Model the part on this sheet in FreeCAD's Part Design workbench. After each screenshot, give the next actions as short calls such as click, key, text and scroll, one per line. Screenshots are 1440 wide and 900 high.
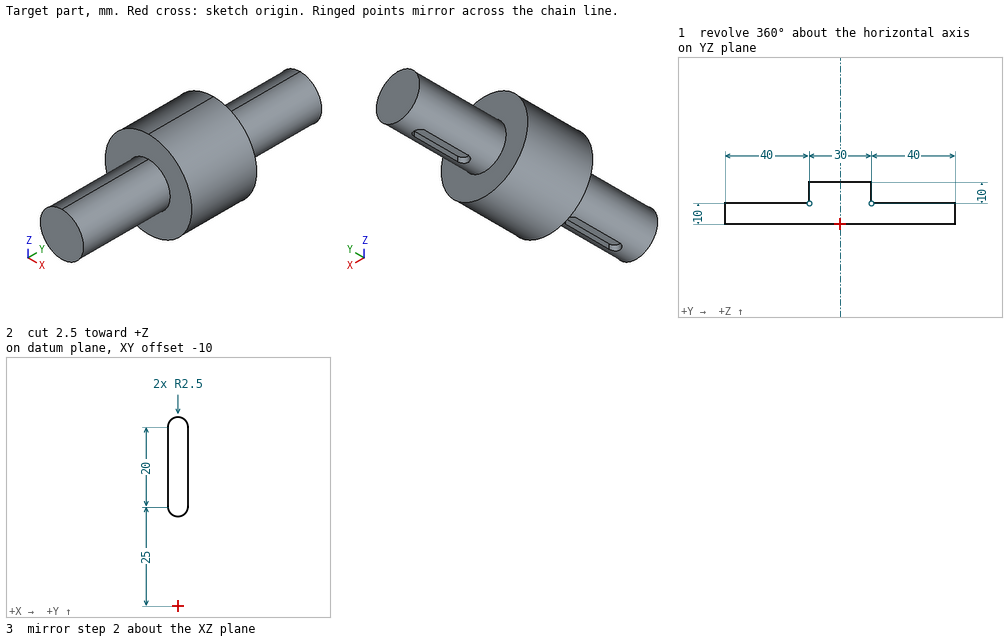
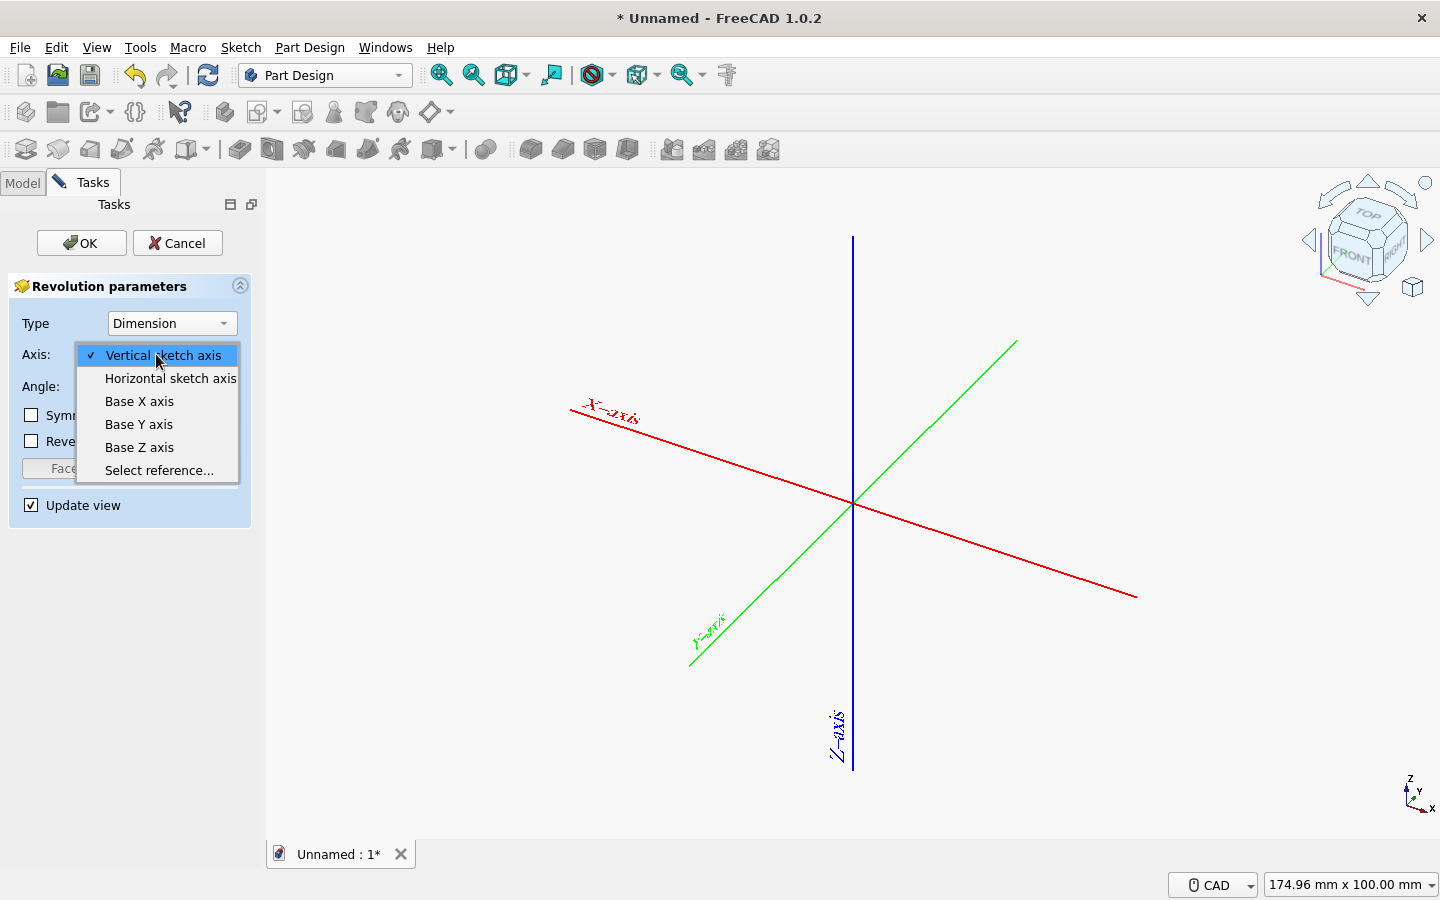
click(156, 378)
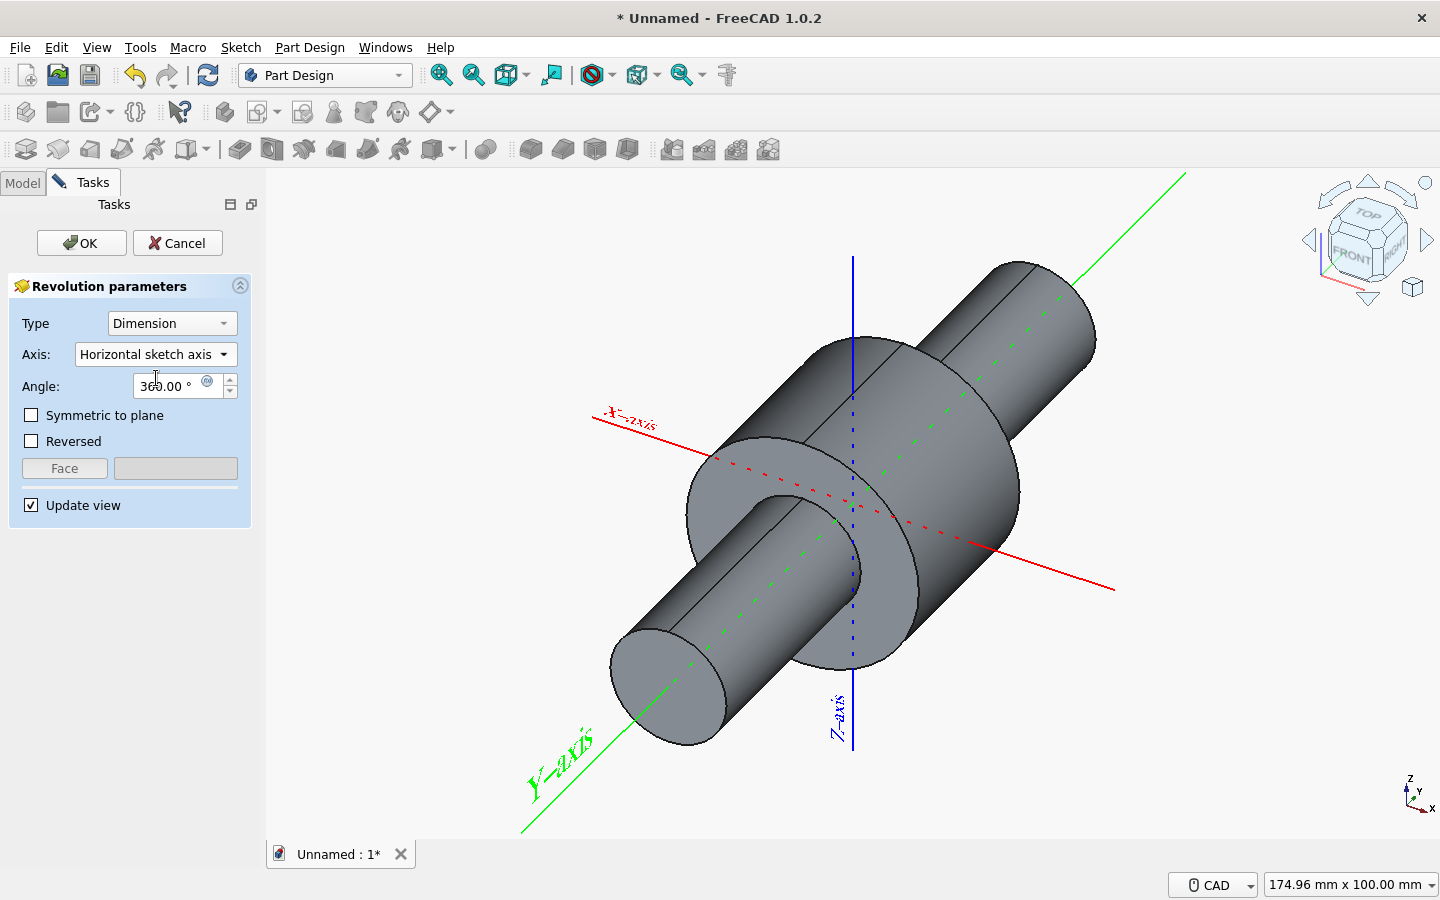
click(82, 243)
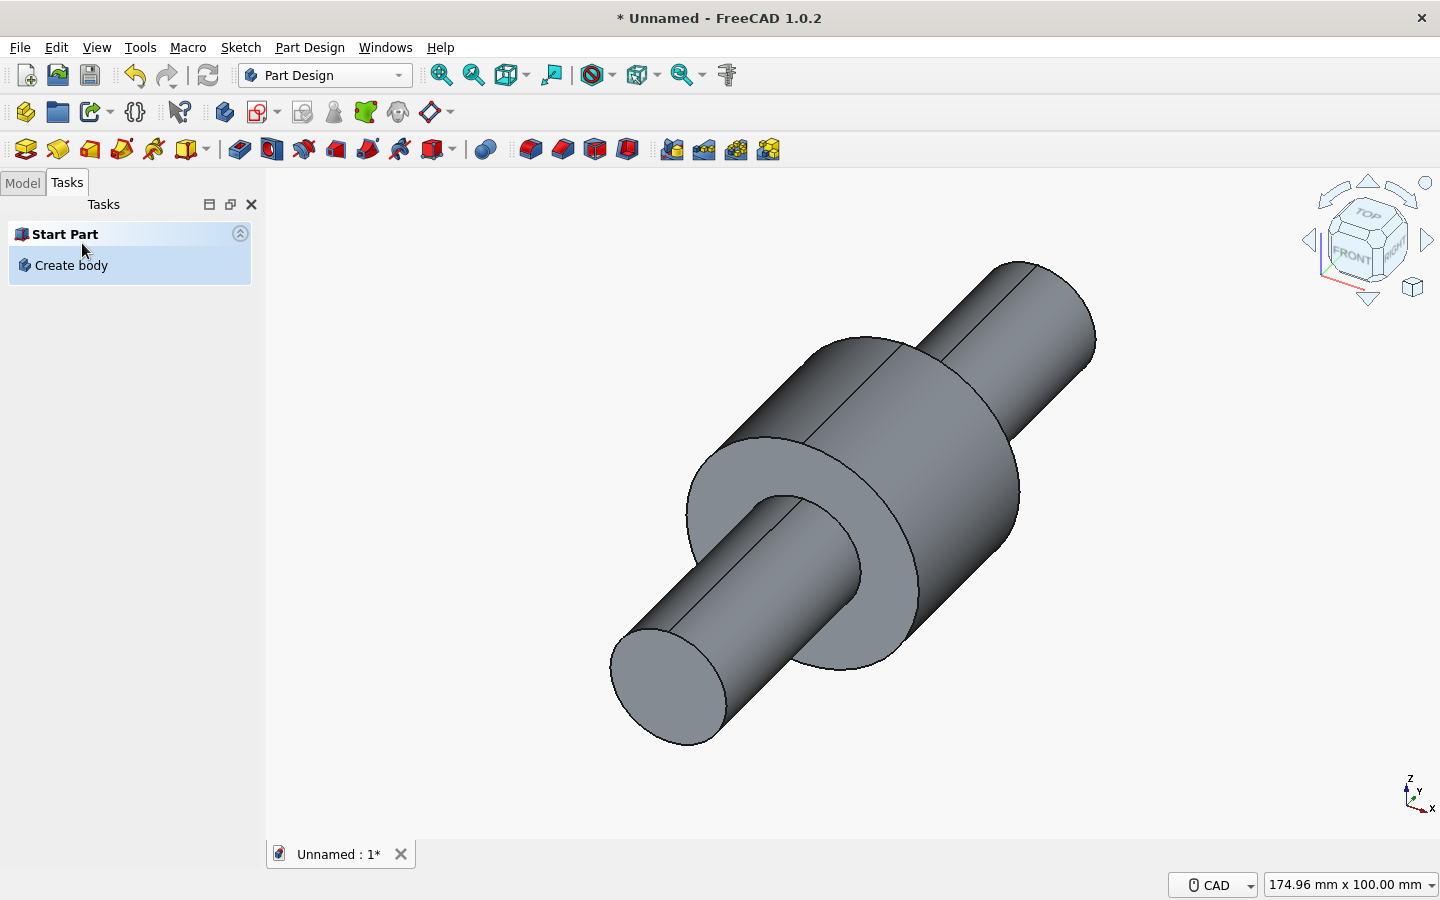
click(23, 182)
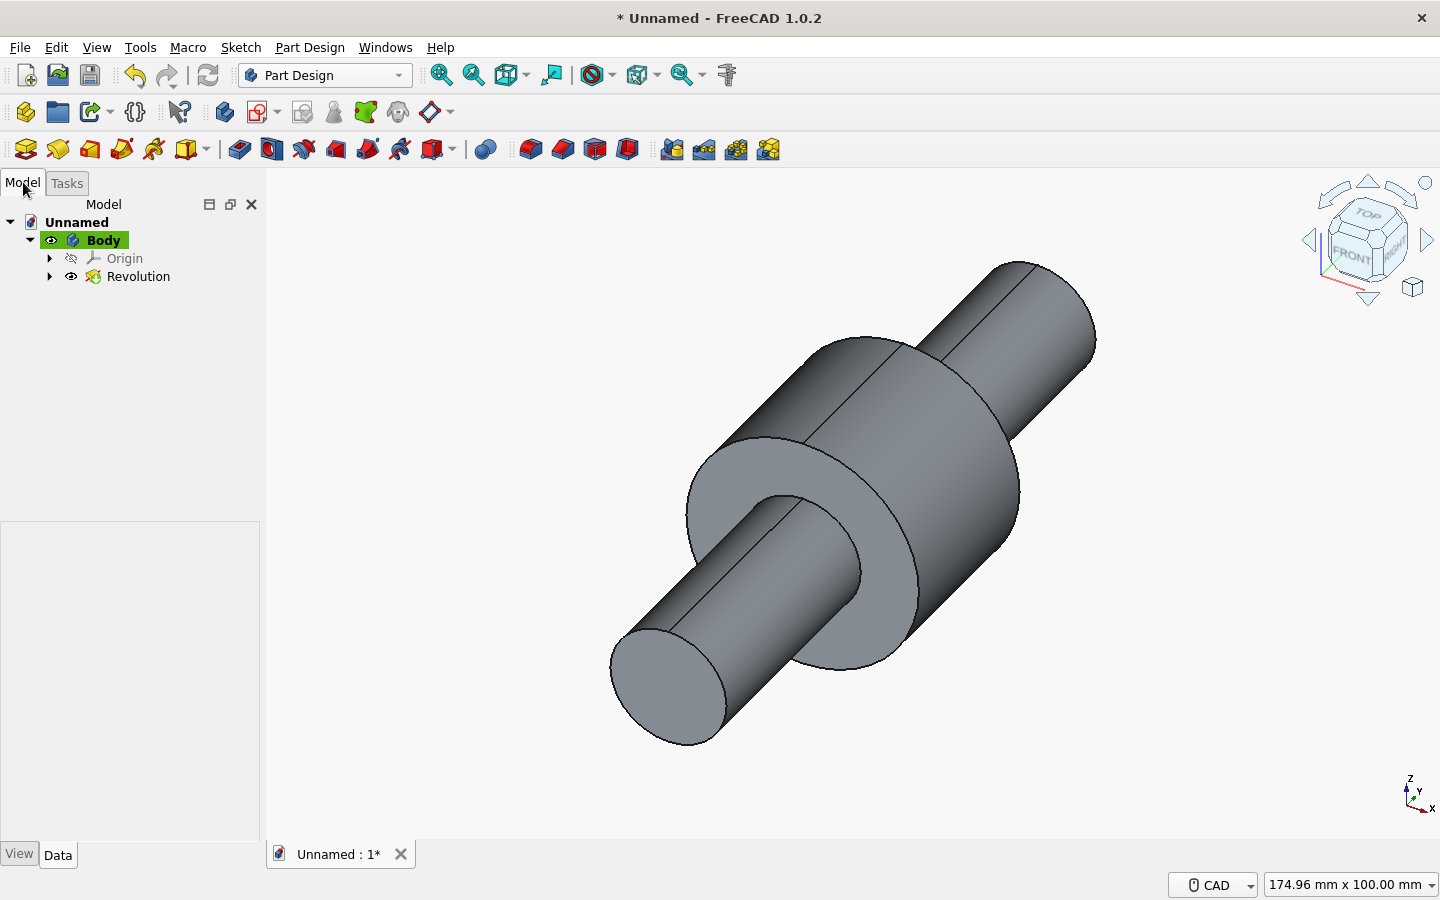
click(50, 258)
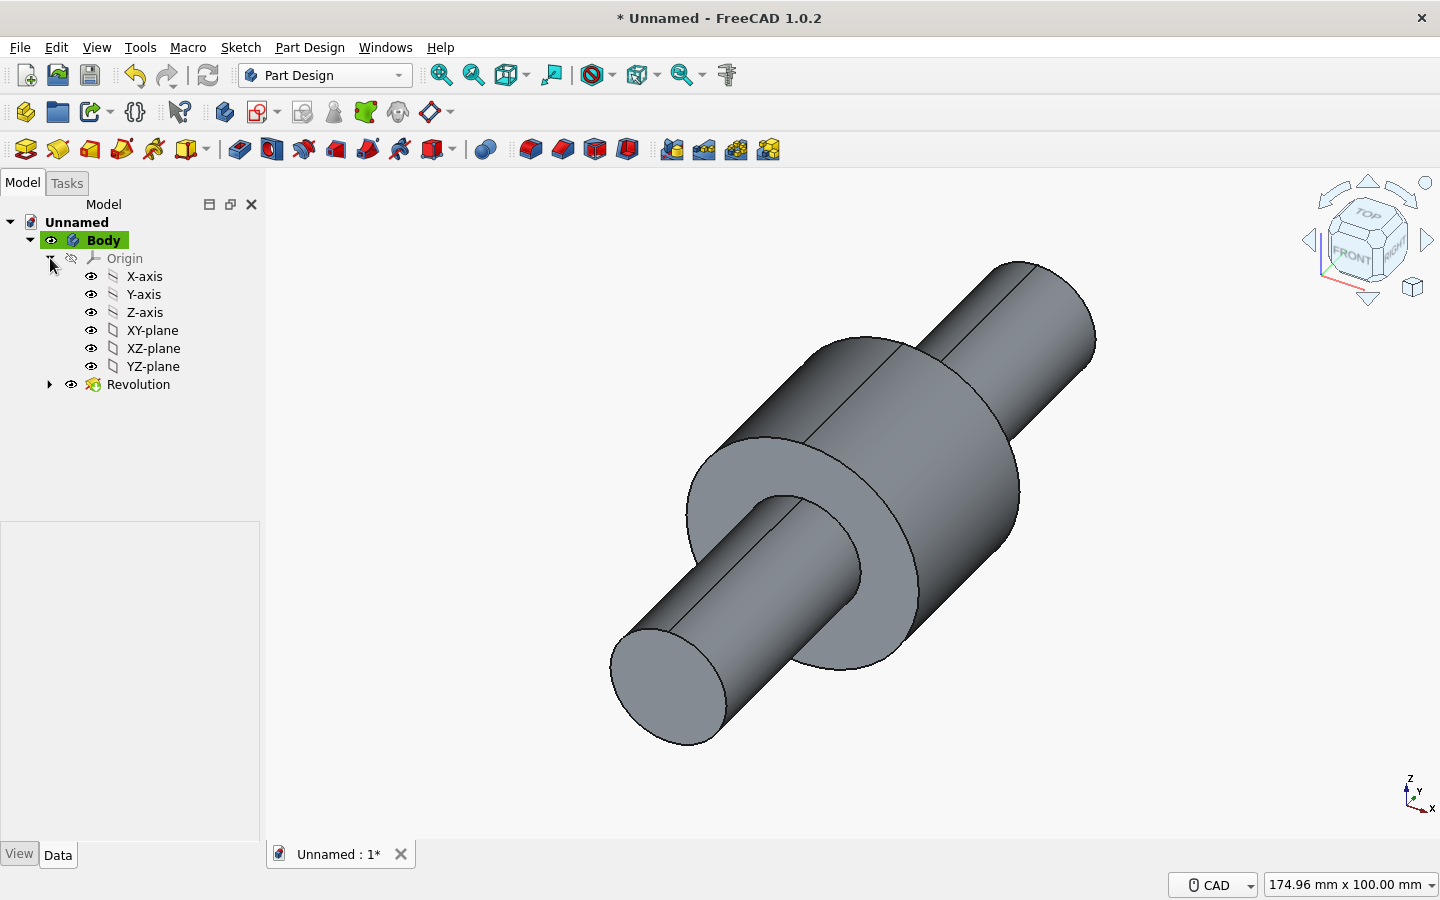
click(136, 330)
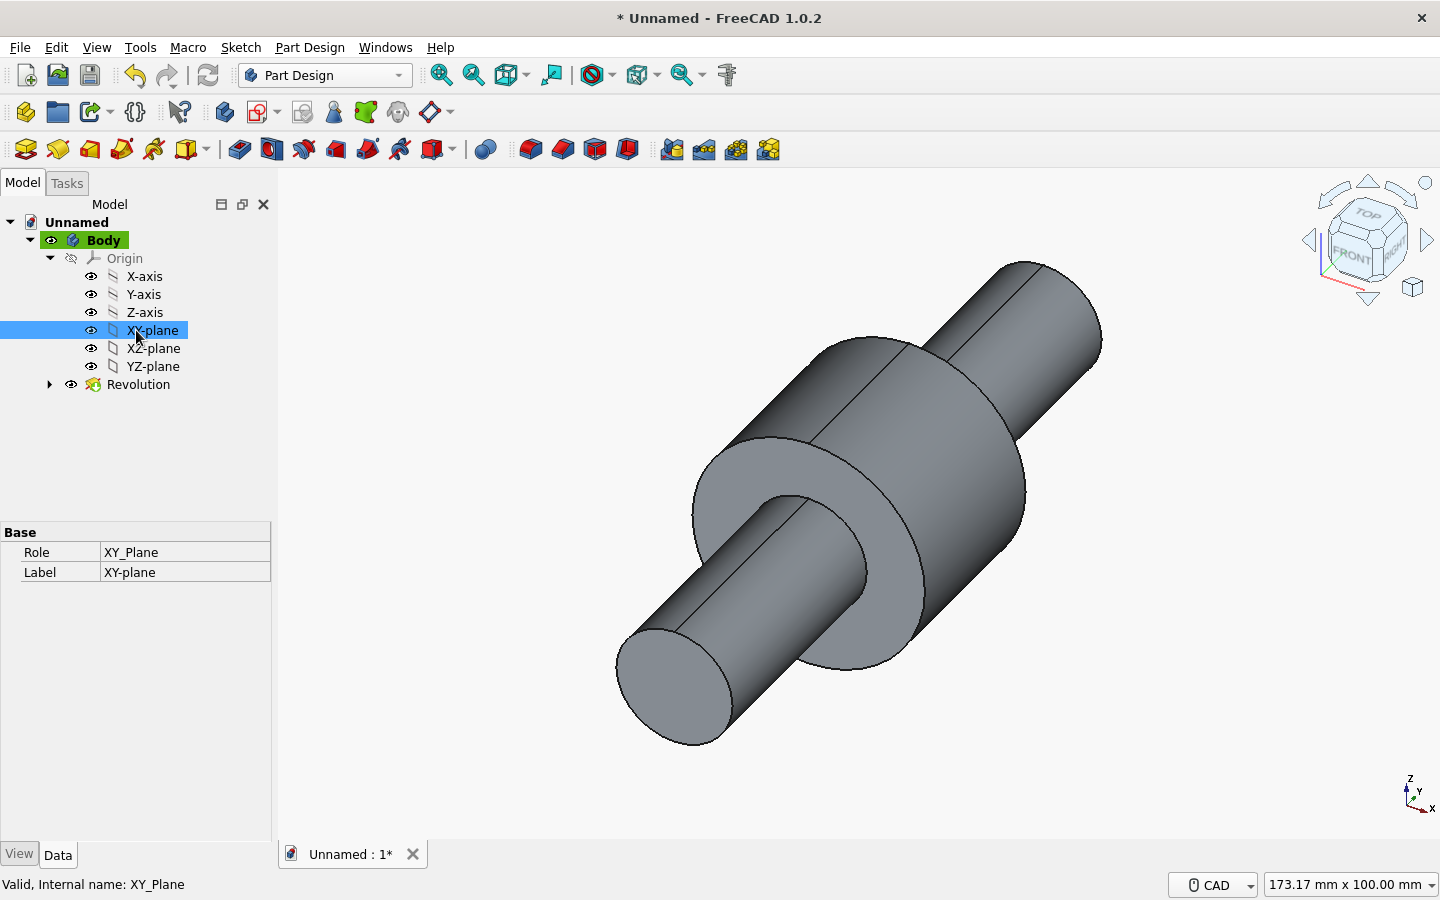
click(430, 112)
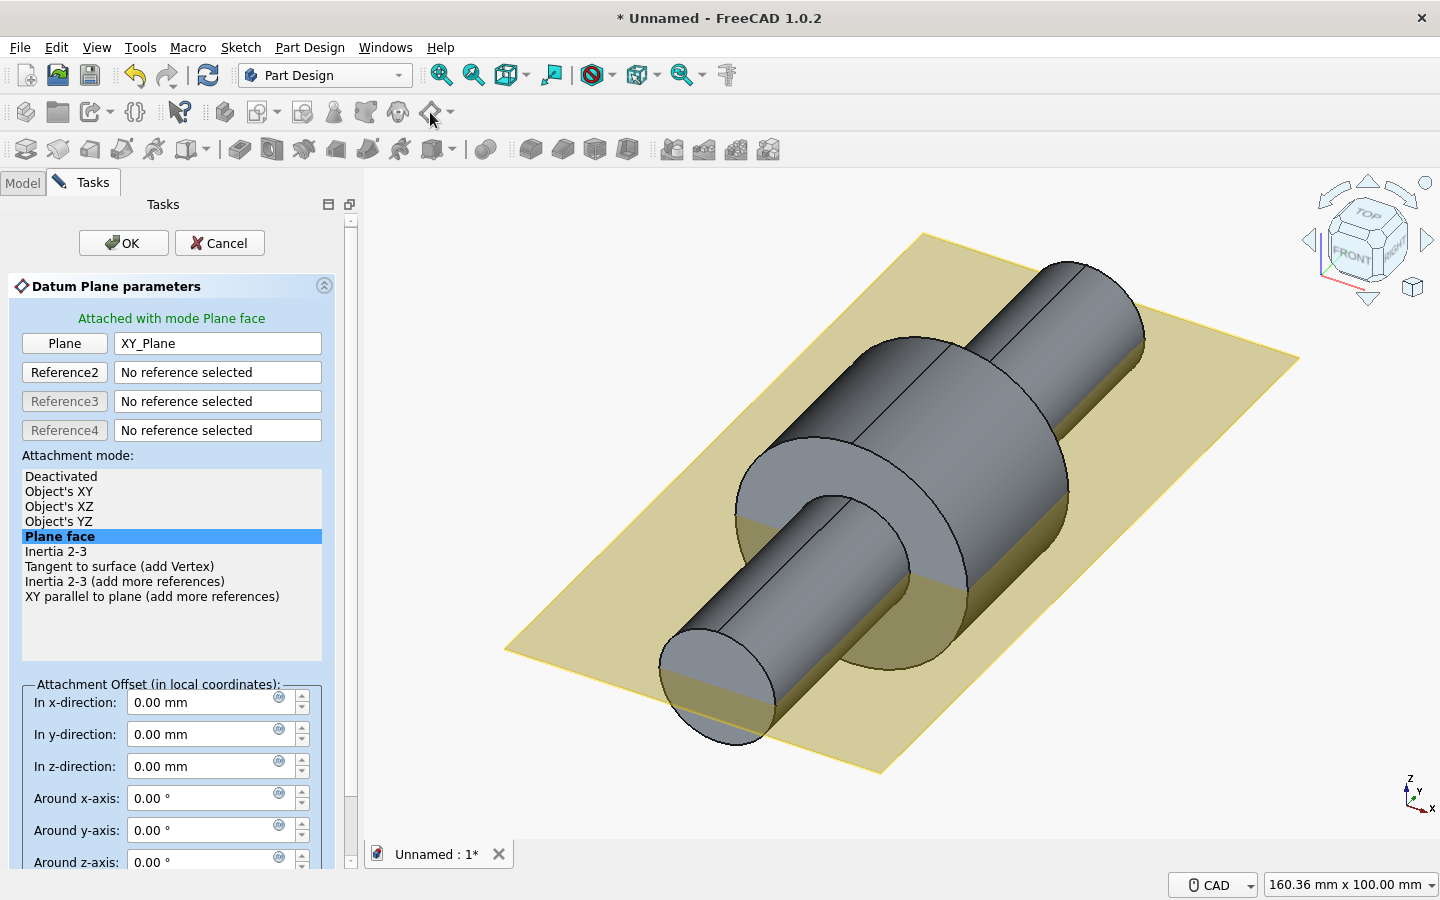
triple_click(210, 766)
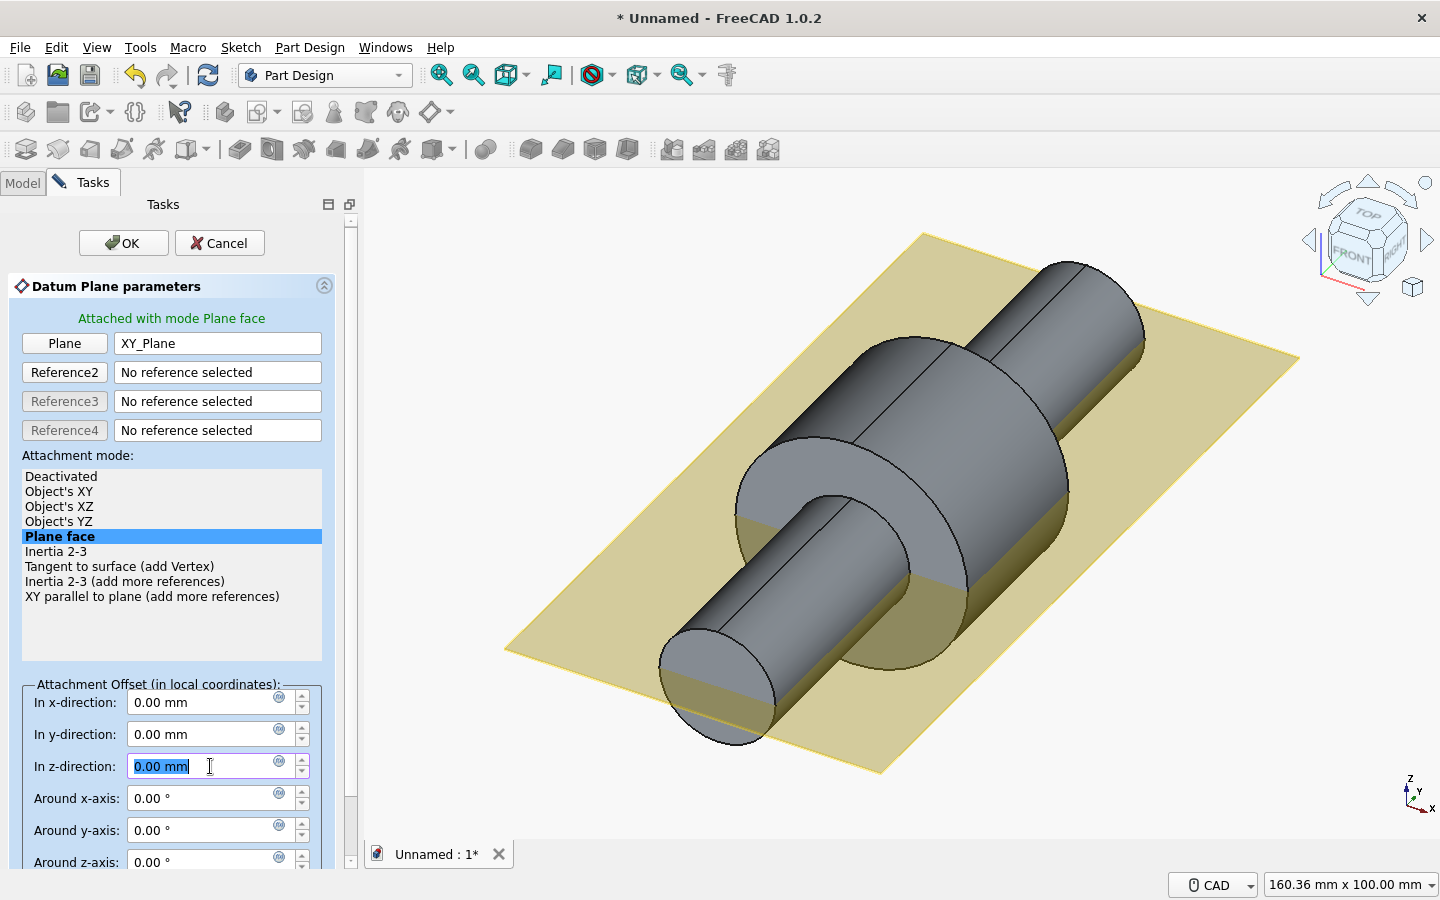
text(-10)
key(Tab)